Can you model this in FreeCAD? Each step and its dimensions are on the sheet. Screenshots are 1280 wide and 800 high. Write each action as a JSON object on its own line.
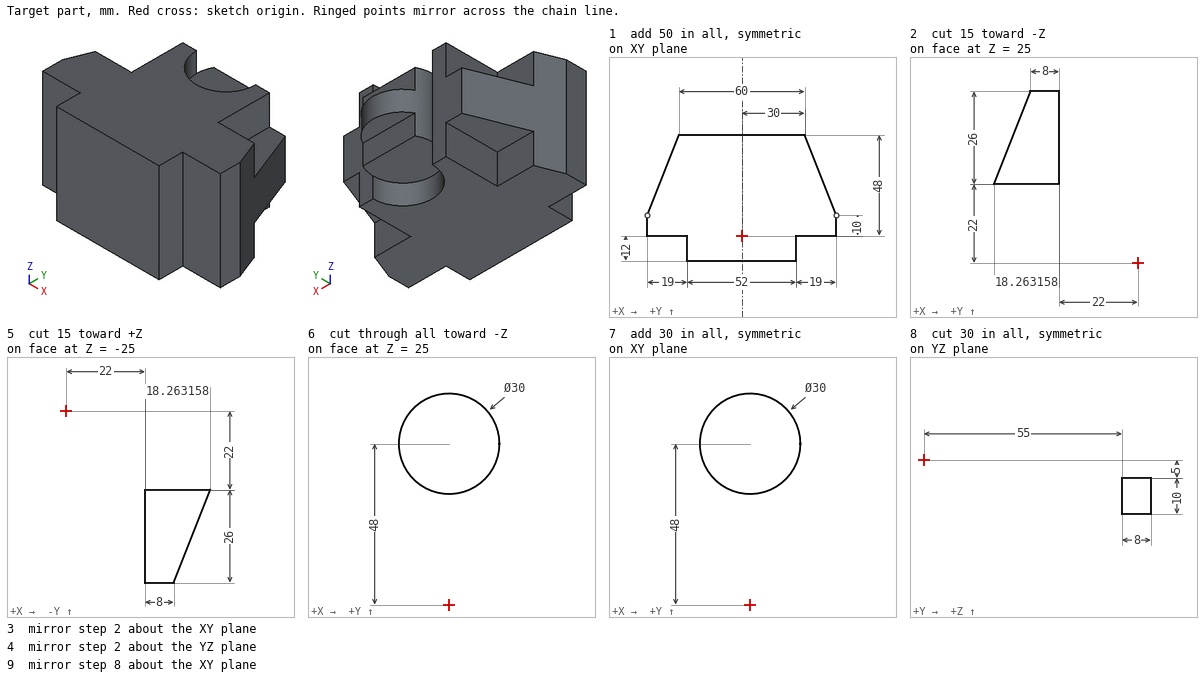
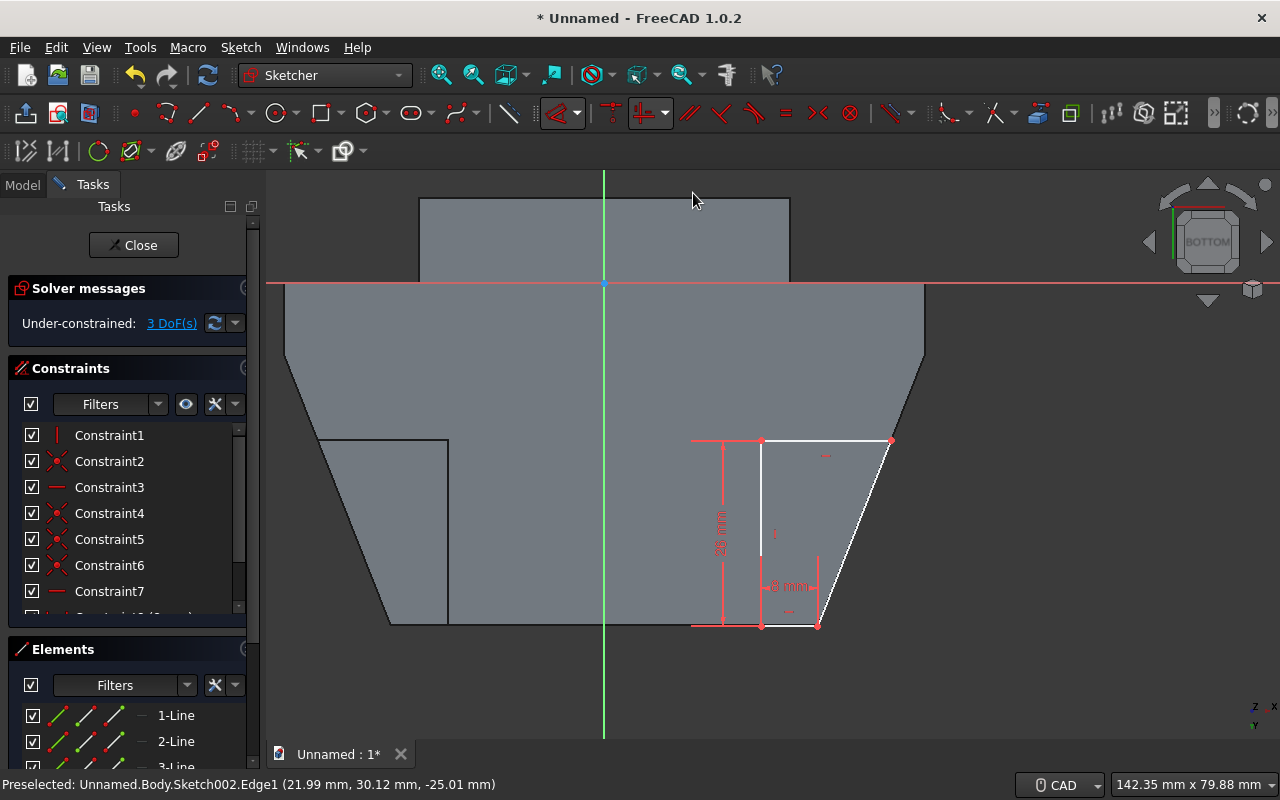
{"action": "left_click", "coordinate": [761, 441]}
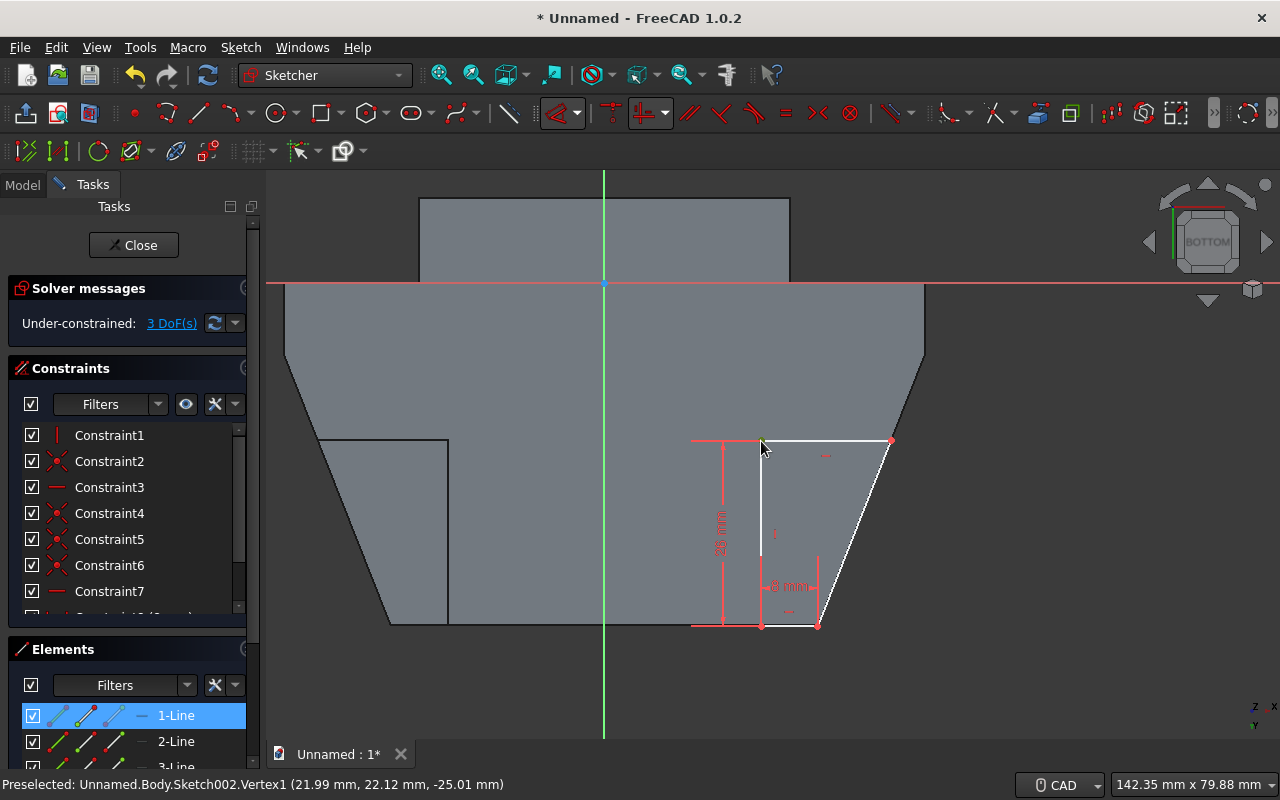
{"action": "left_click", "coordinate": [580, 114]}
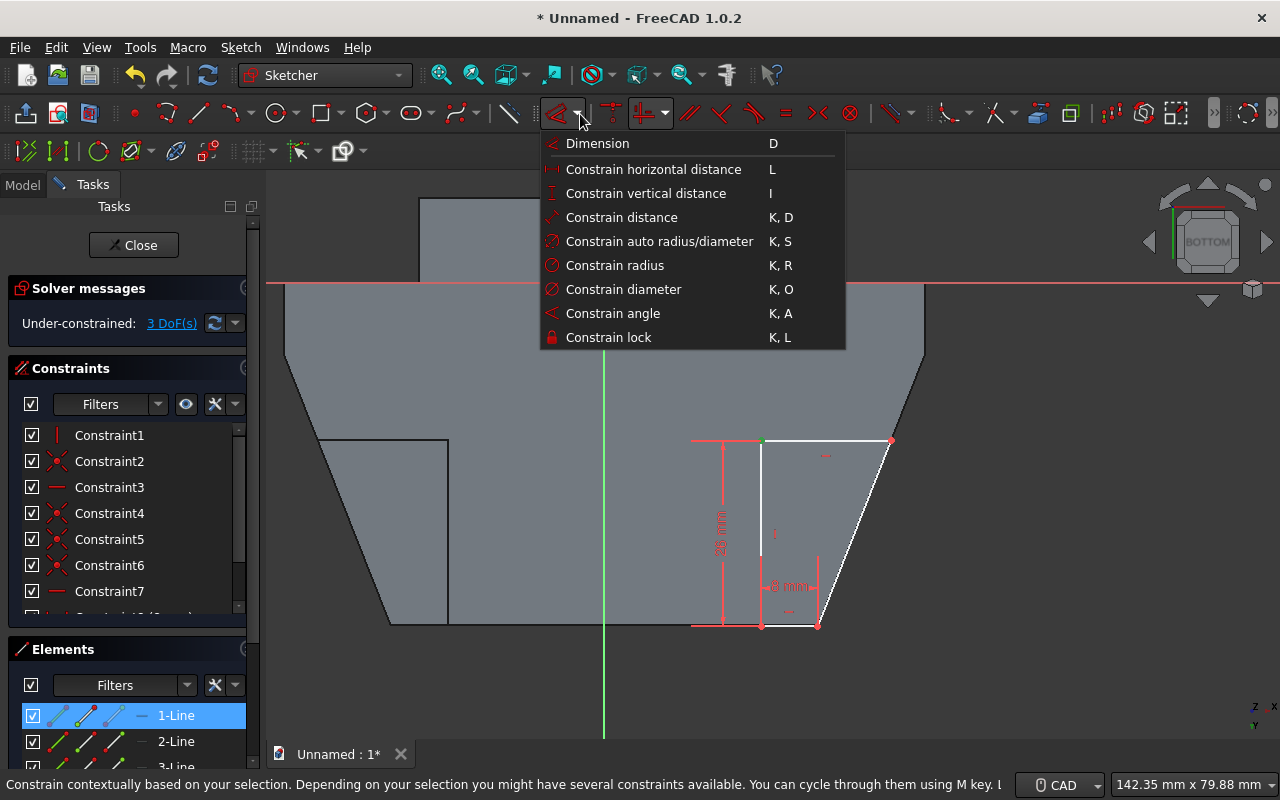
{"action": "left_click", "coordinate": [693, 169]}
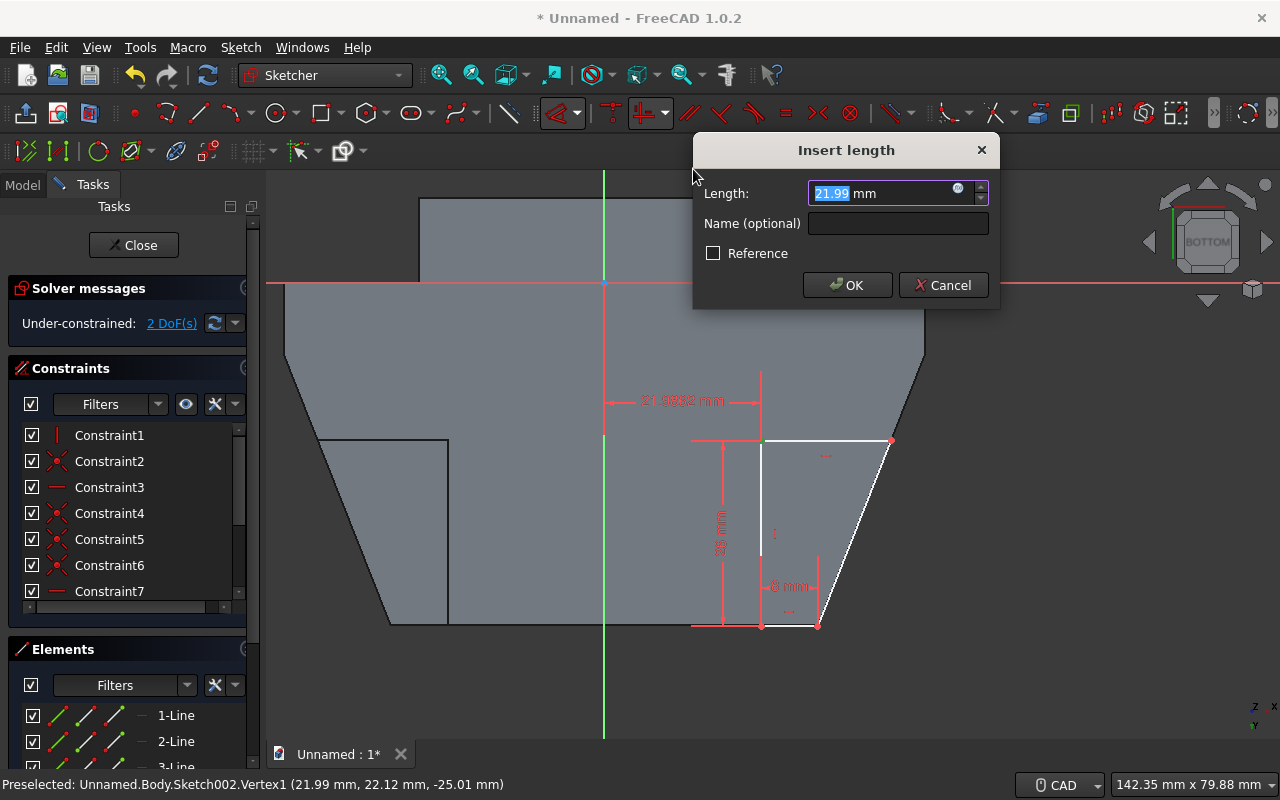
{"action": "type", "text": "22"}
{"action": "key", "text": "Return"}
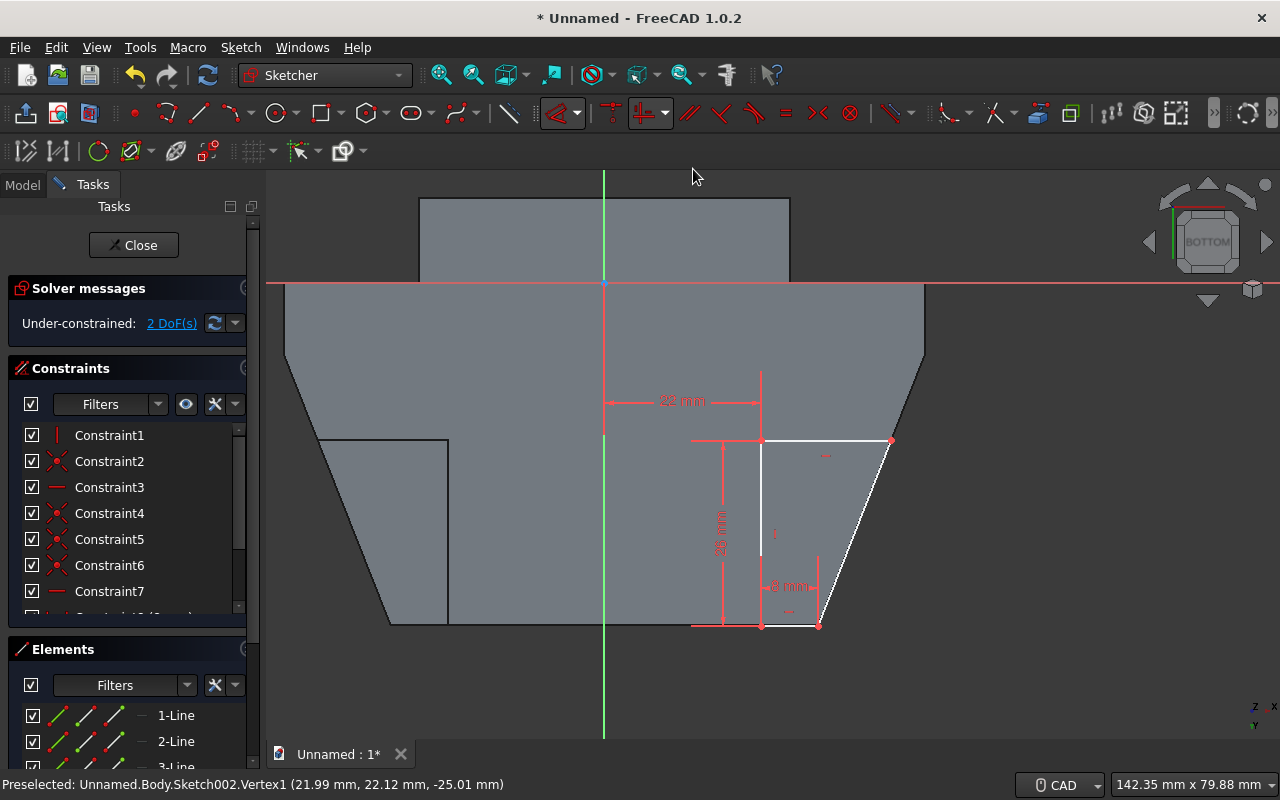
{"action": "left_click", "coordinate": [761, 441]}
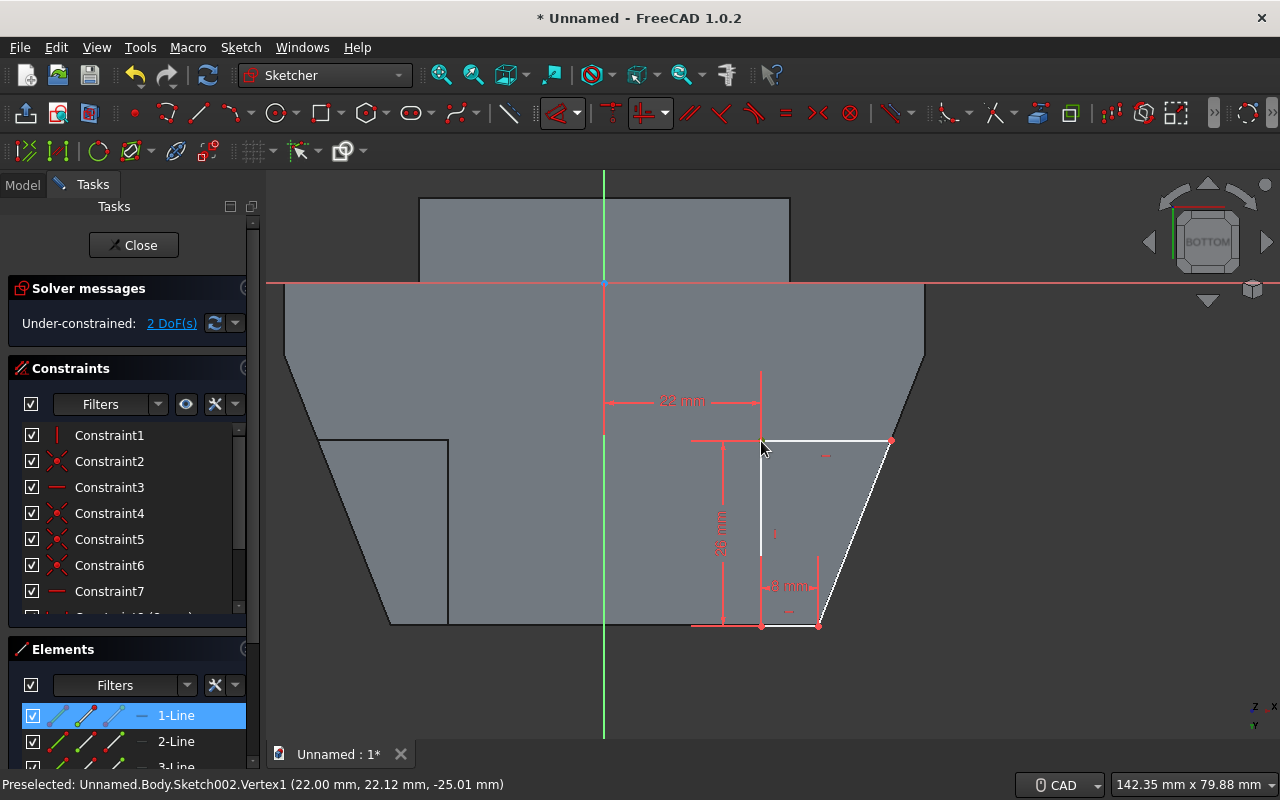
{"action": "key", "text": "i"}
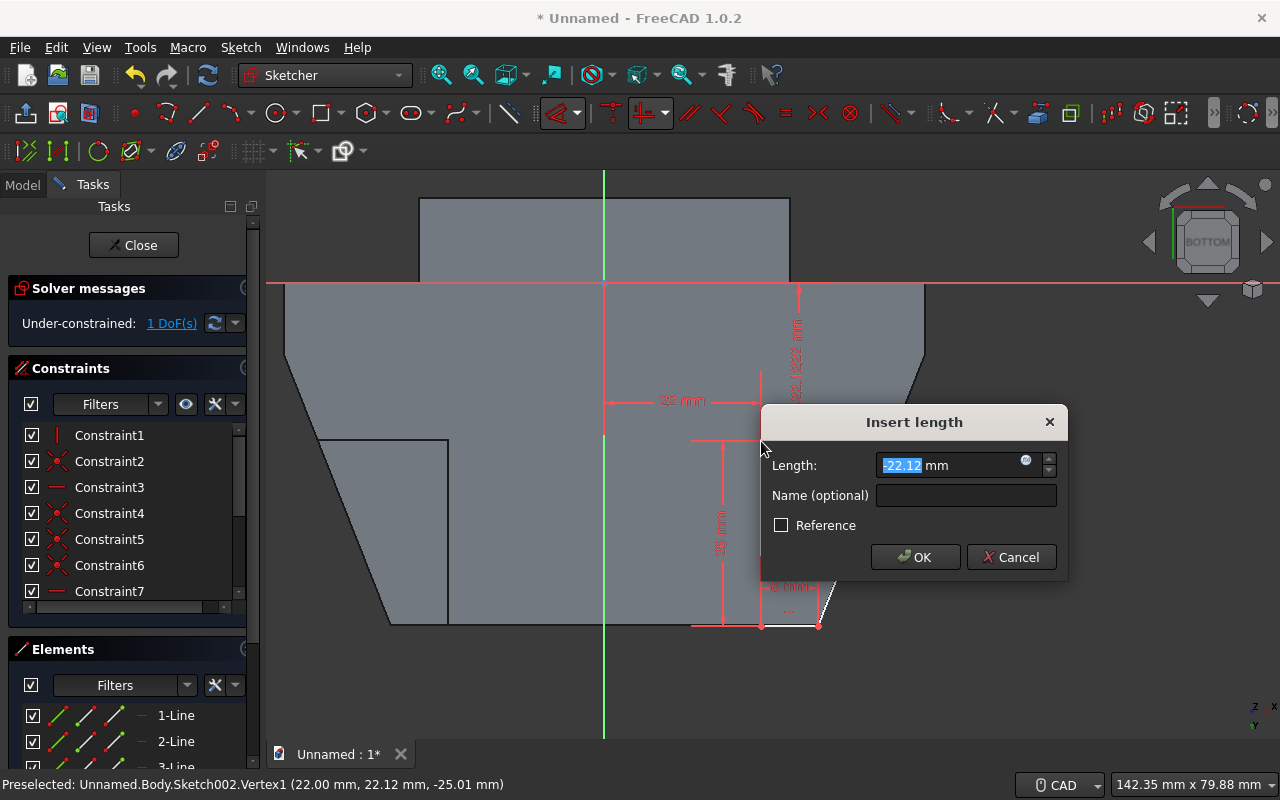
{"action": "type", "text": "-22"}
{"action": "key", "text": "Return"}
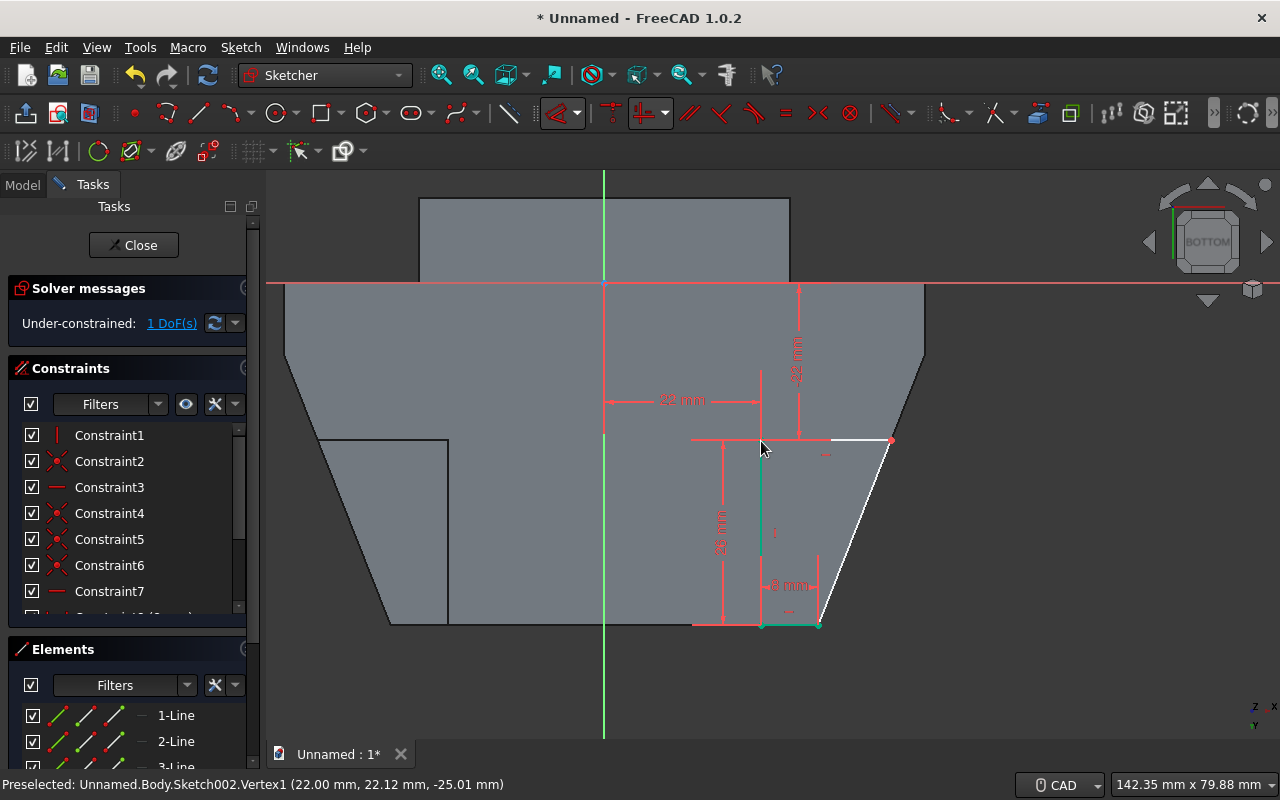
{"action": "left_click", "coordinate": [852, 440]}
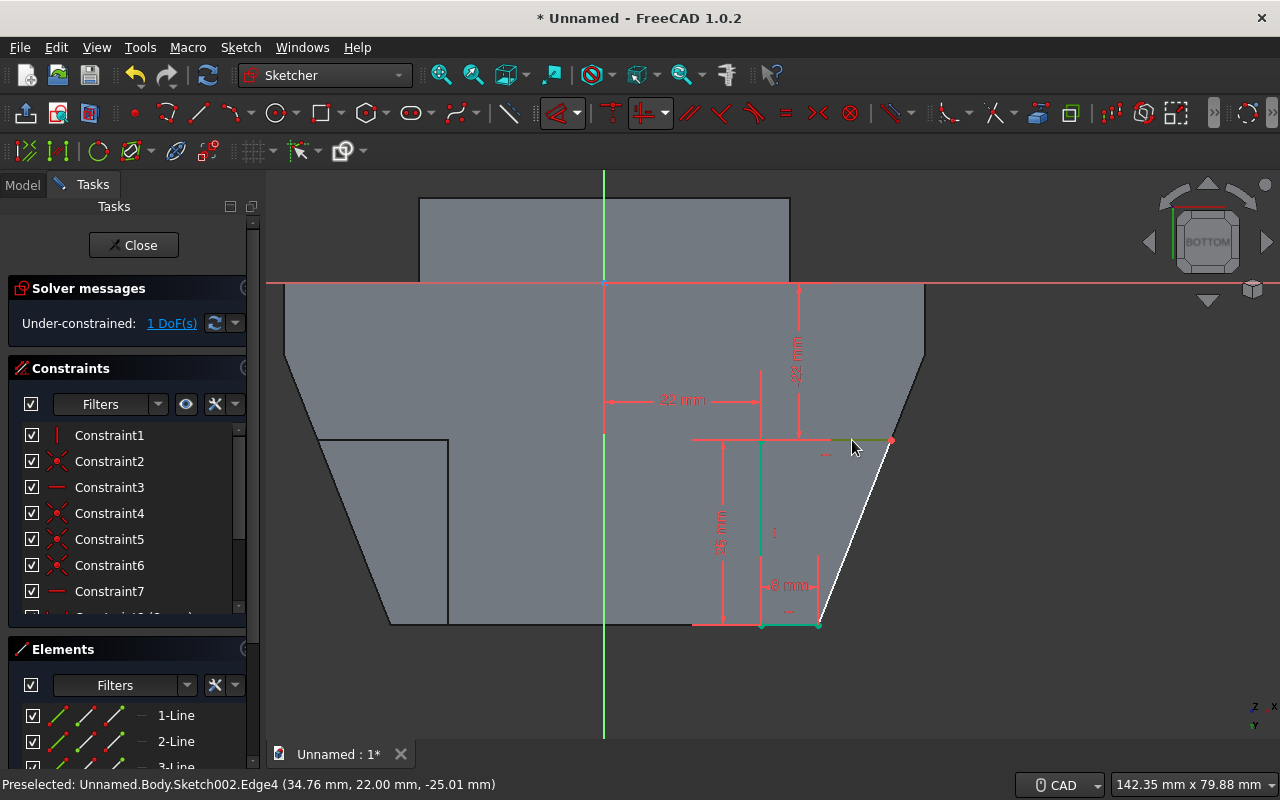
{"action": "key", "text": "l"}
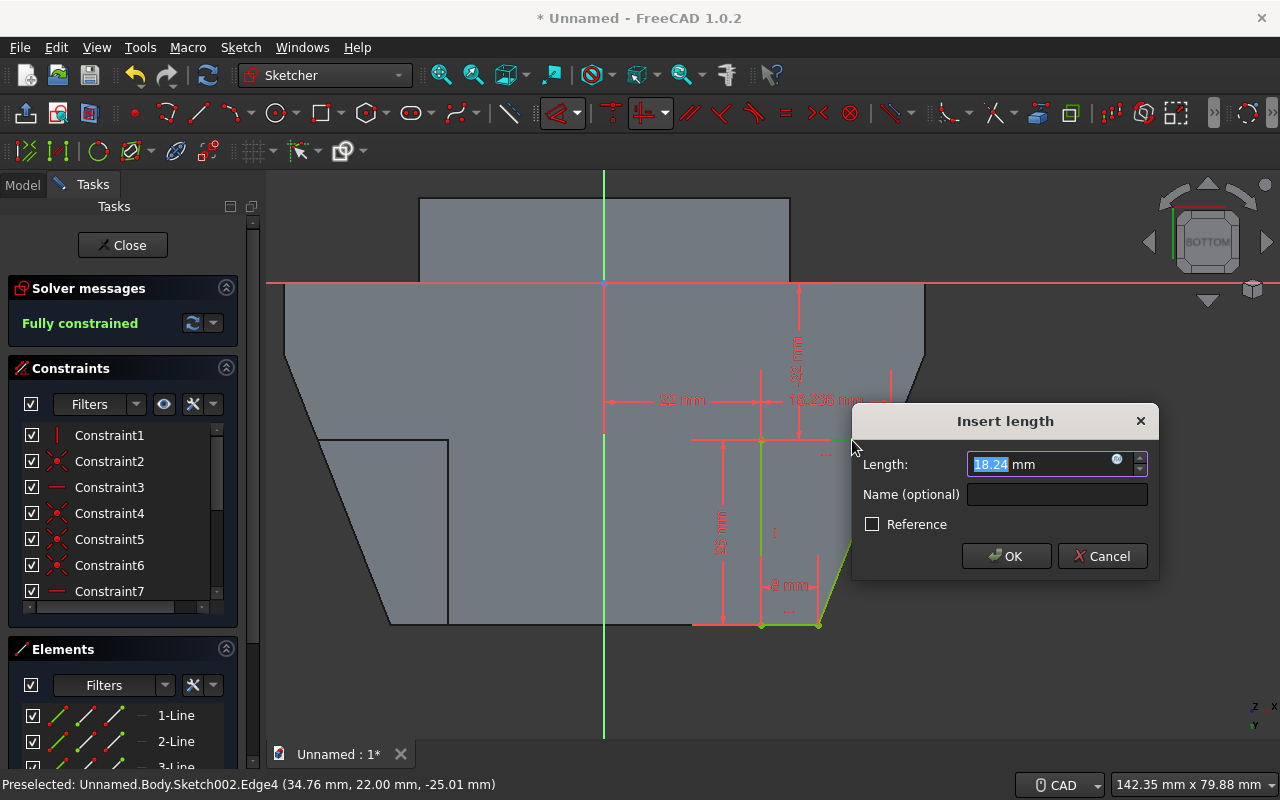
{"action": "type", "text": "18.263158"}
{"action": "key", "text": "Return"}